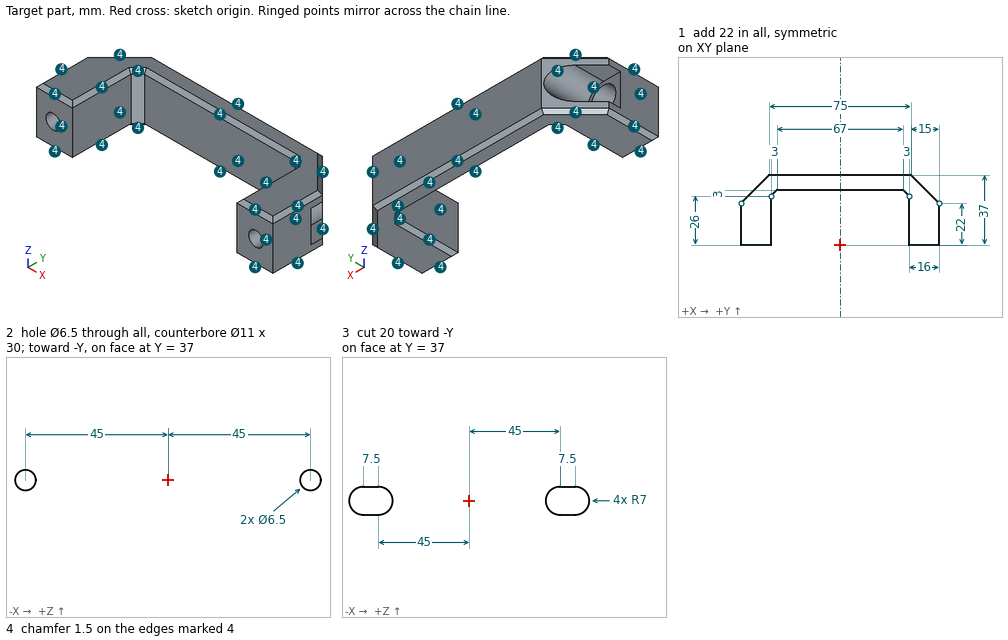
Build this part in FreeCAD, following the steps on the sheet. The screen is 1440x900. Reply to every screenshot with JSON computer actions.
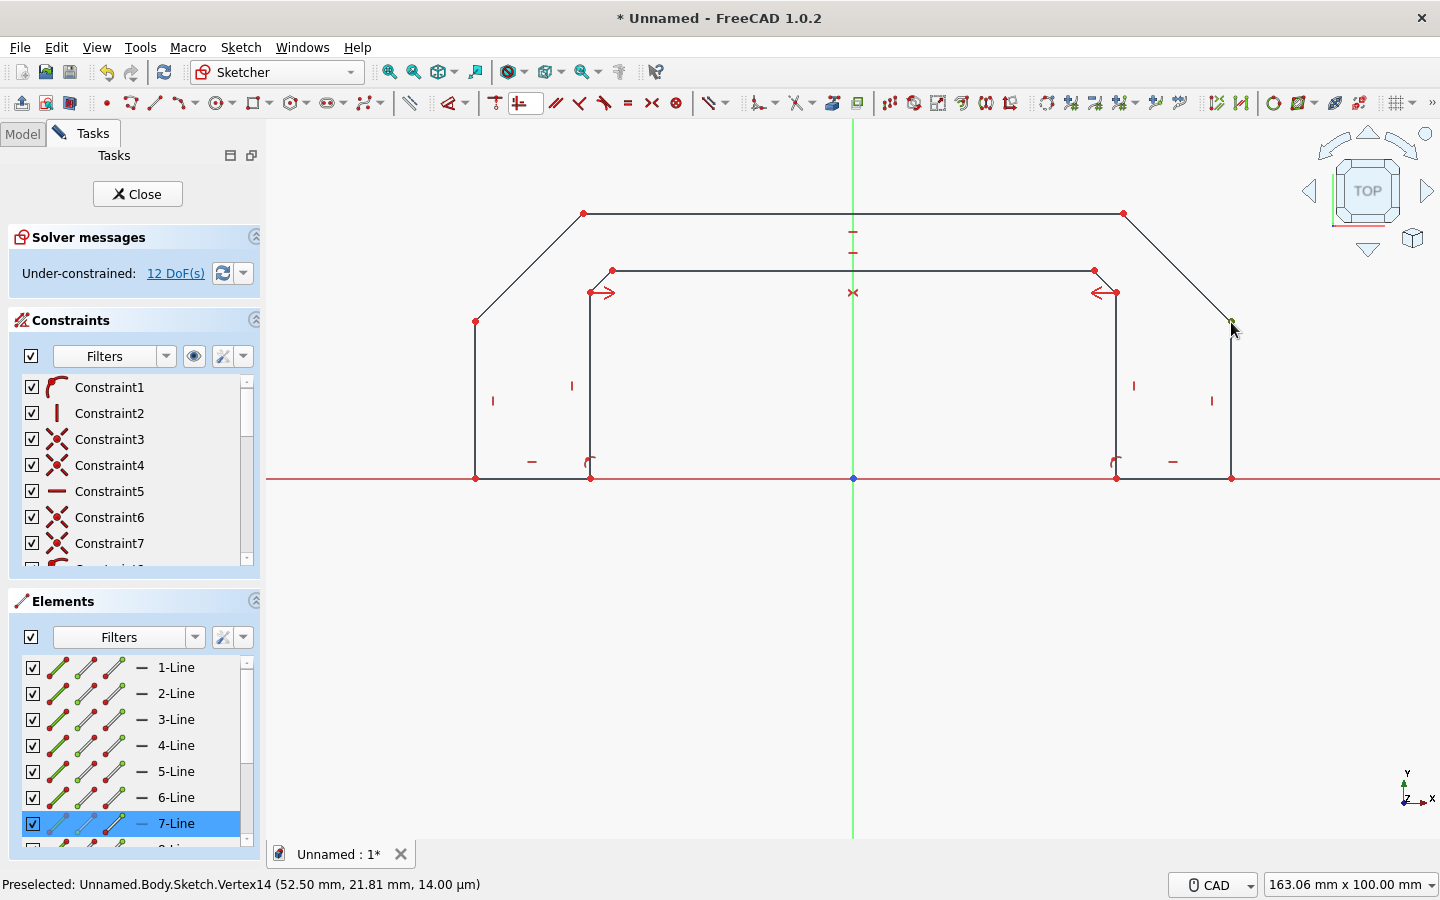
{"action": "left_click", "coordinate": [475, 322]}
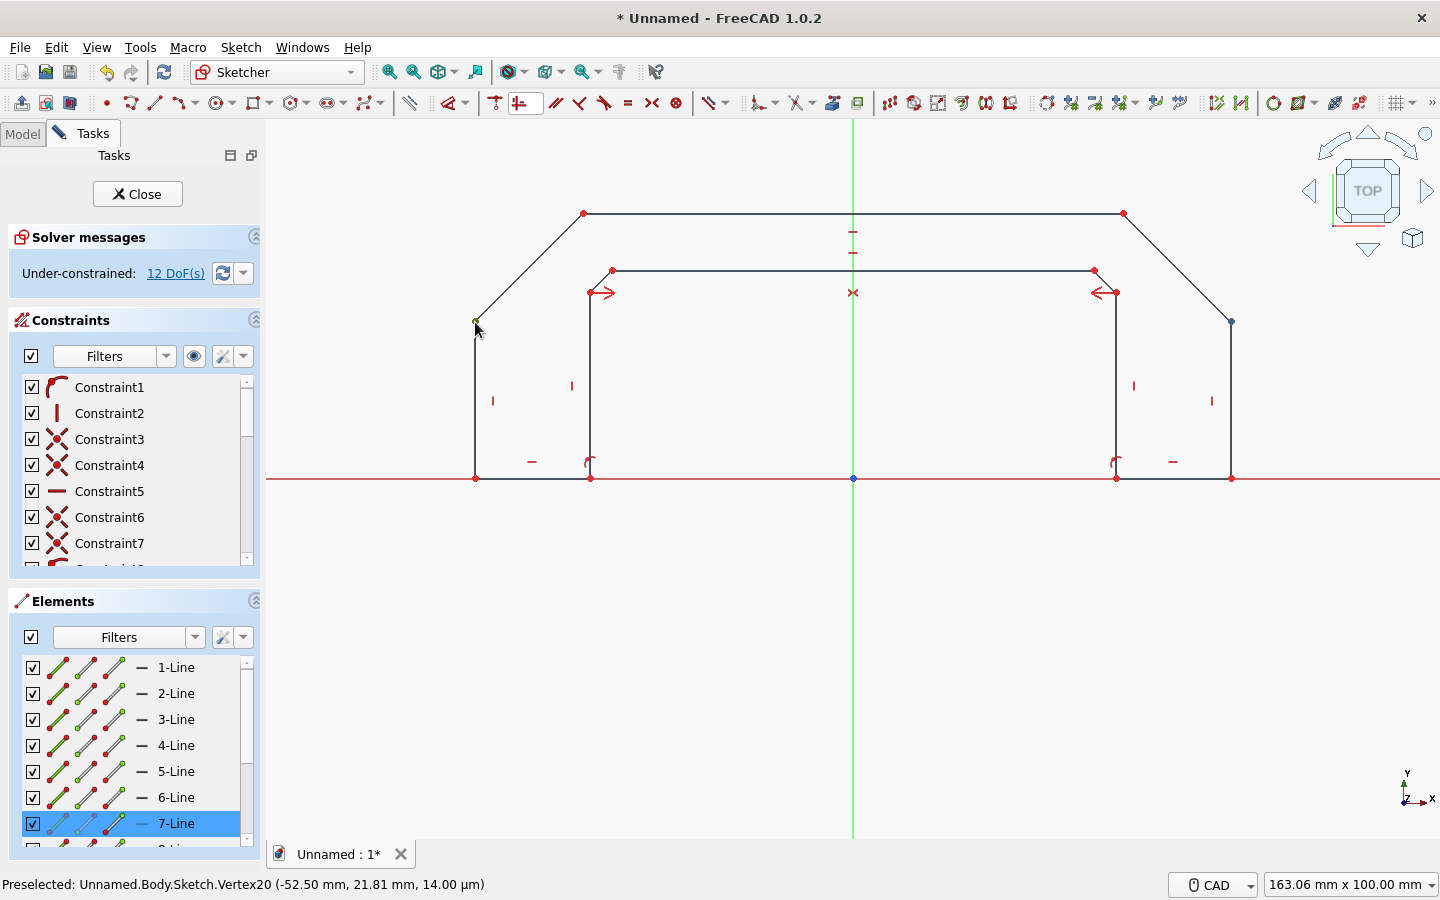
{"action": "left_click", "coordinate": [853, 764]}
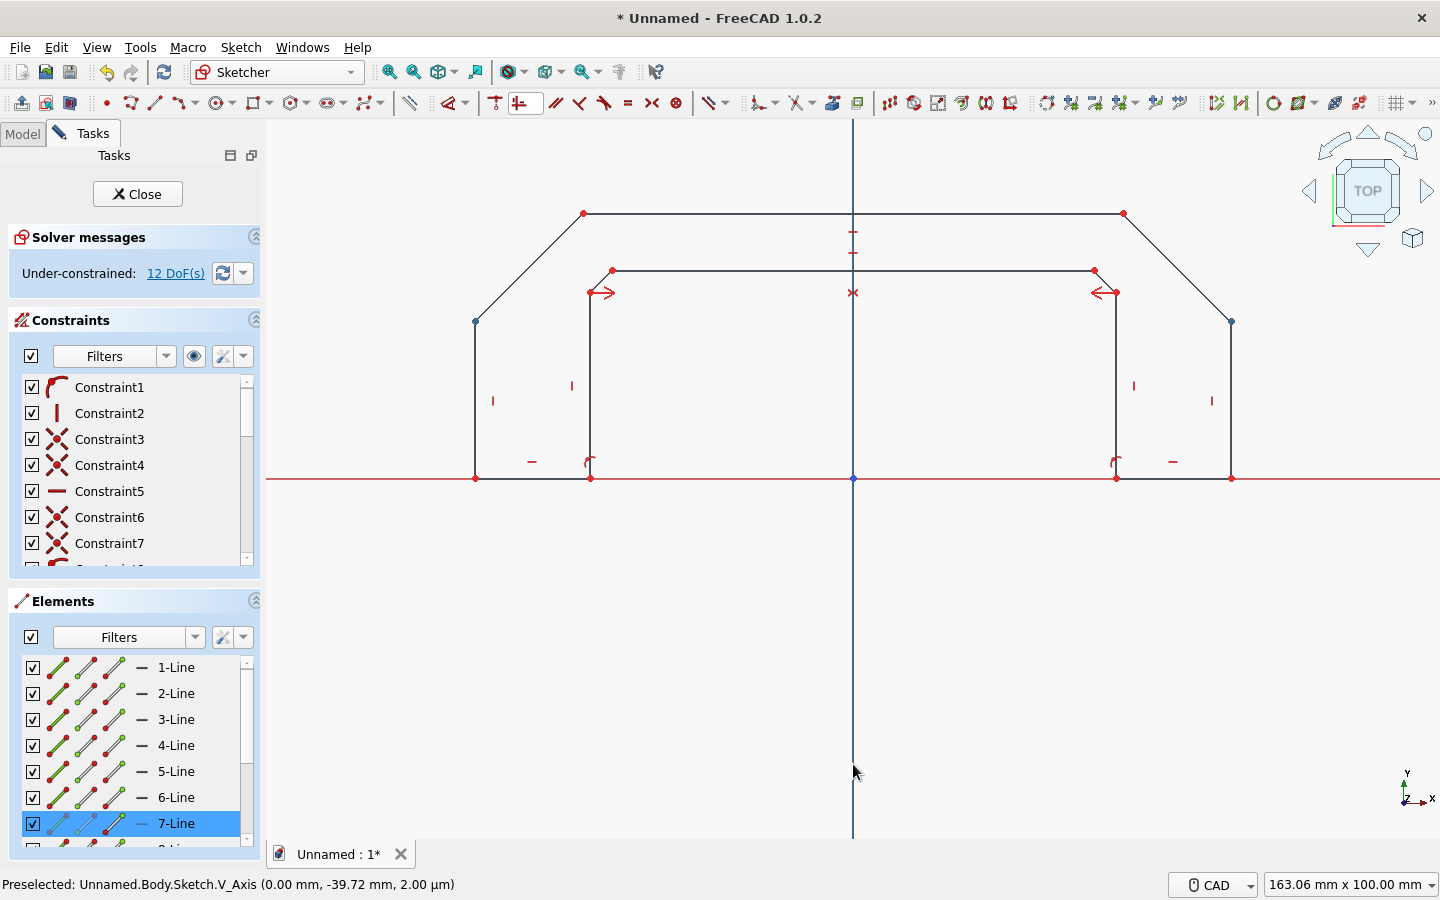
{"action": "left_click", "coordinate": [652, 104]}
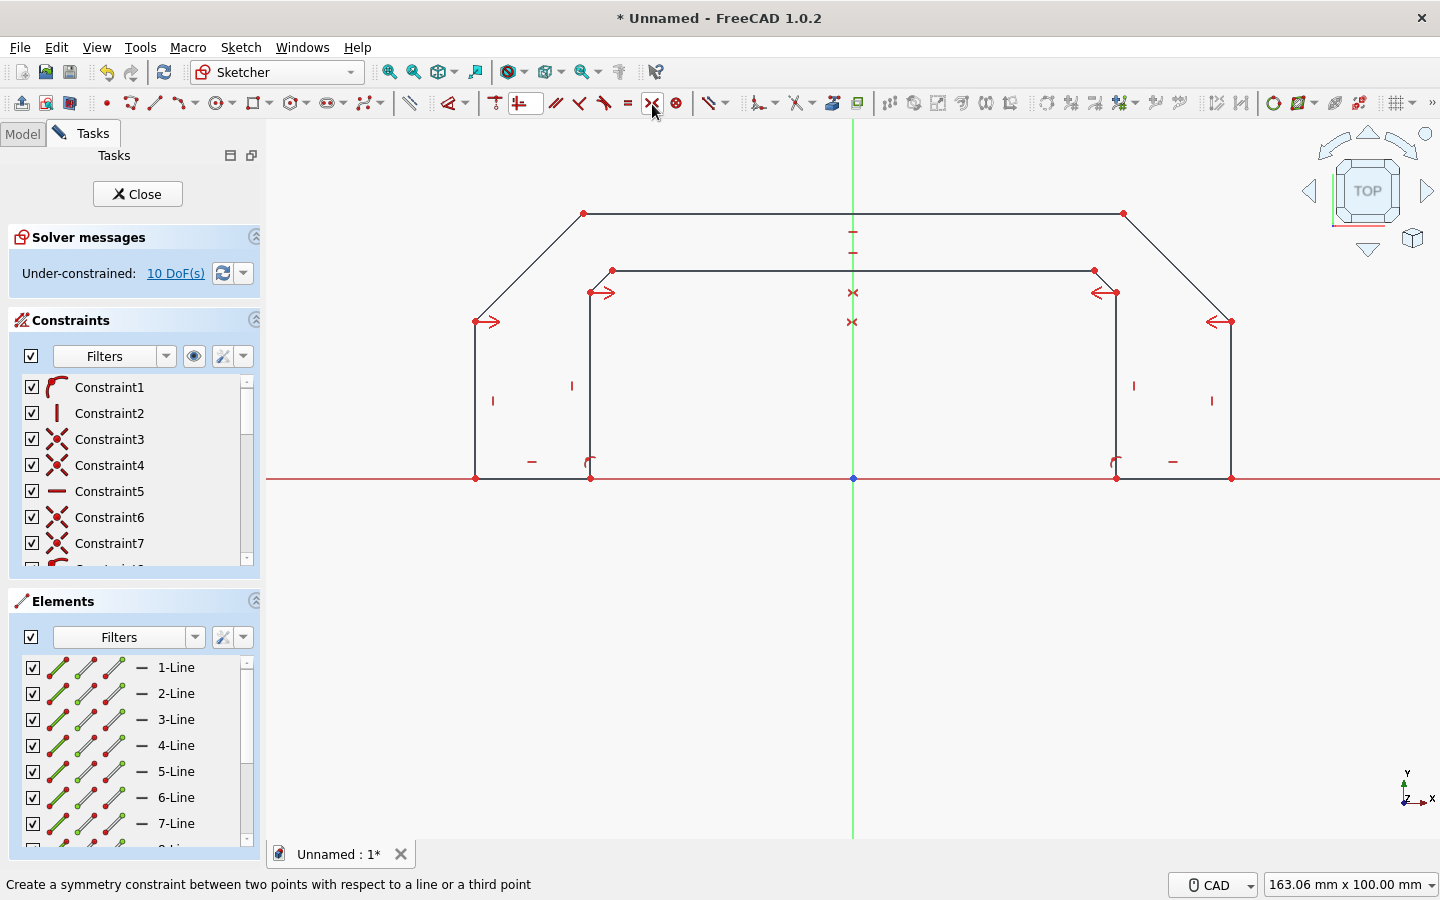
{"action": "left_click", "coordinate": [590, 423]}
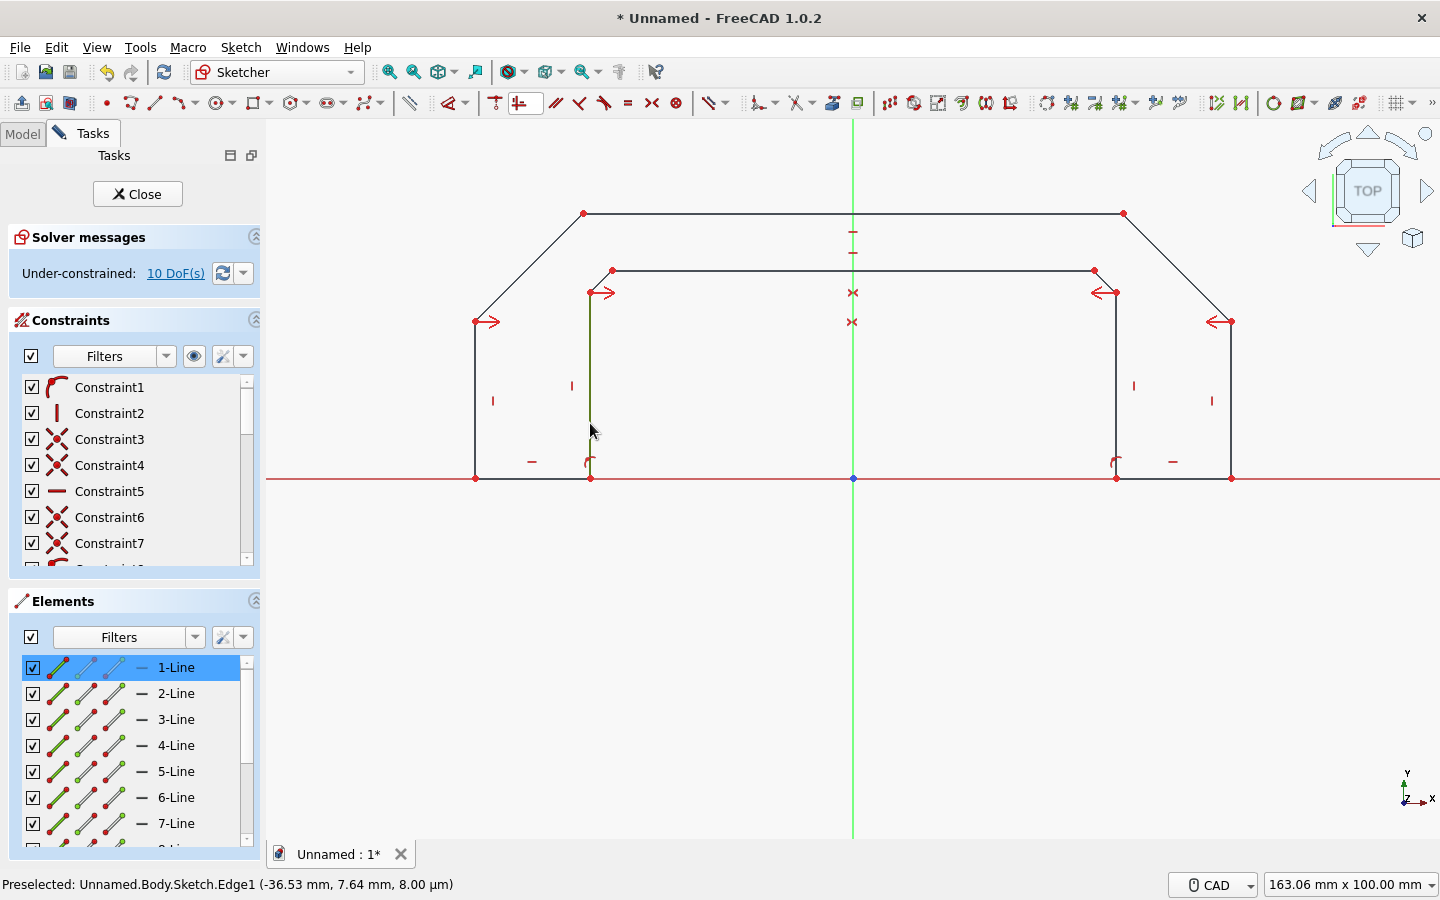
{"action": "left_click", "coordinate": [468, 104]}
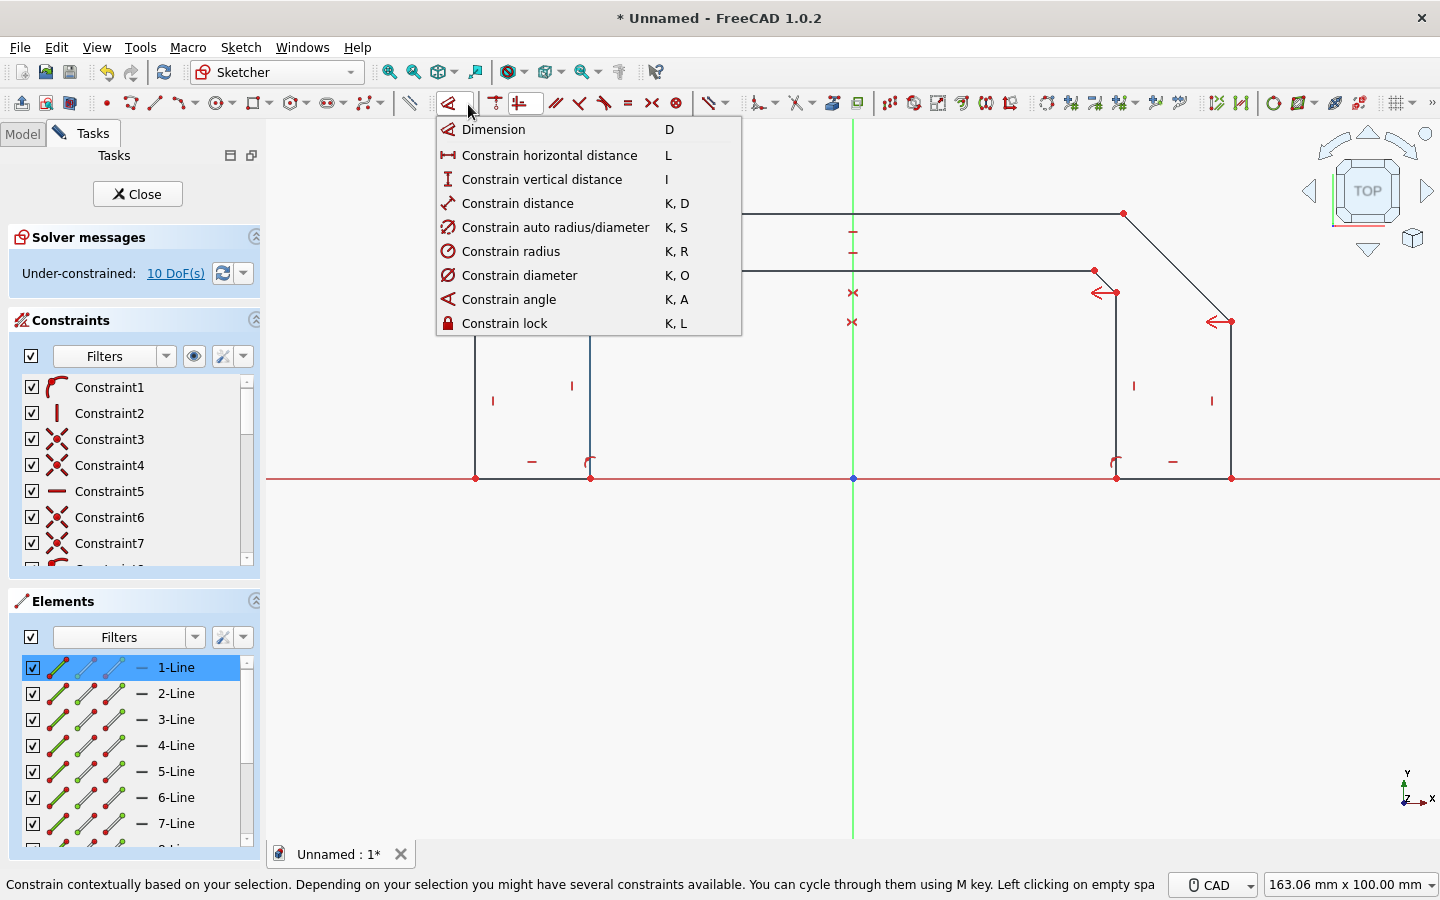
{"action": "left_click", "coordinate": [589, 179]}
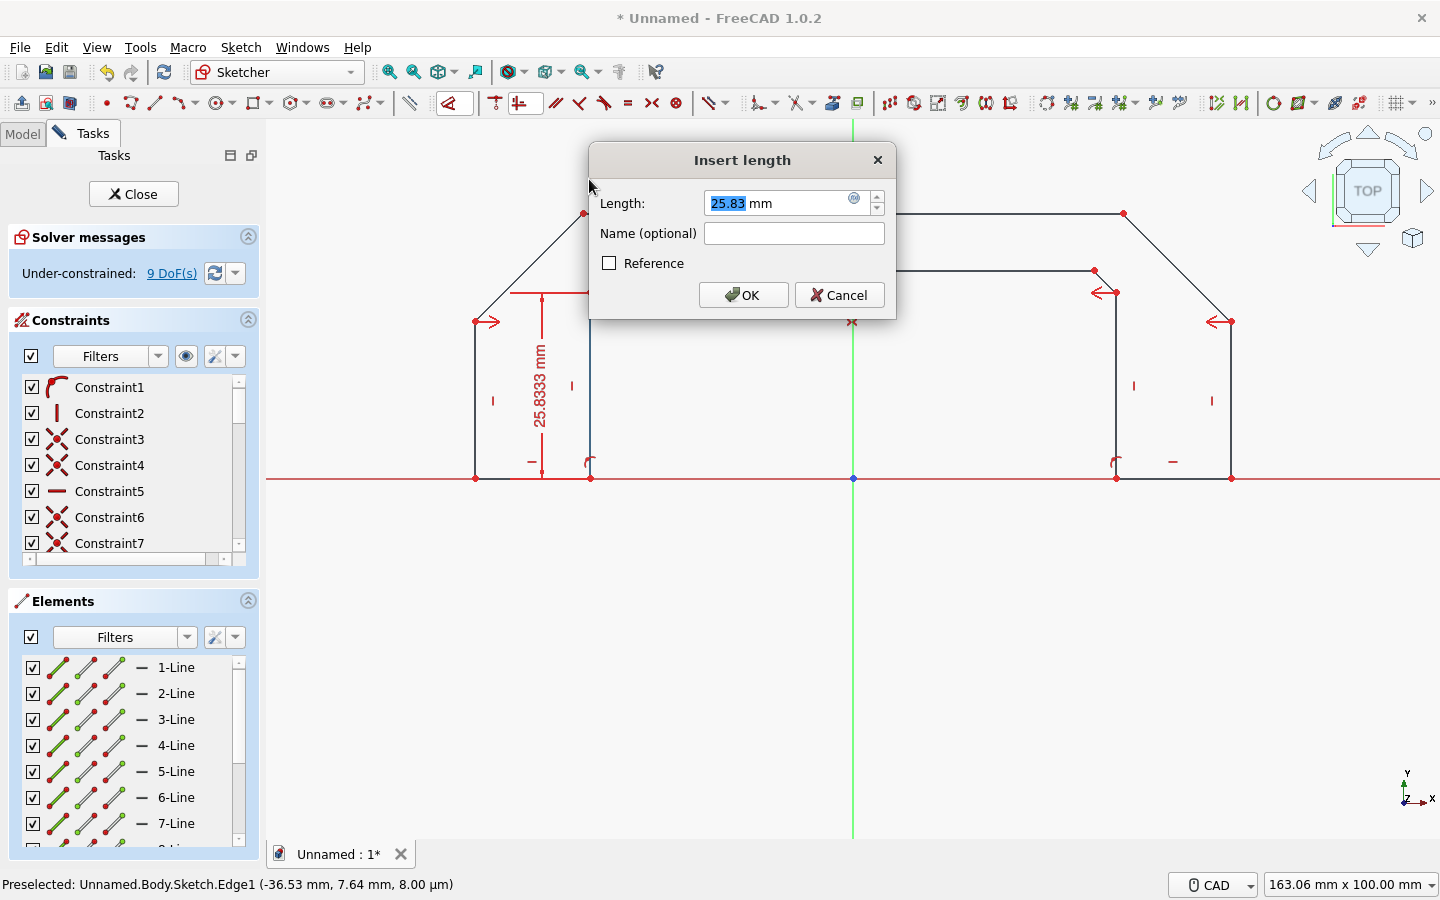
{"action": "type", "text": "26"}
{"action": "key", "text": "Return"}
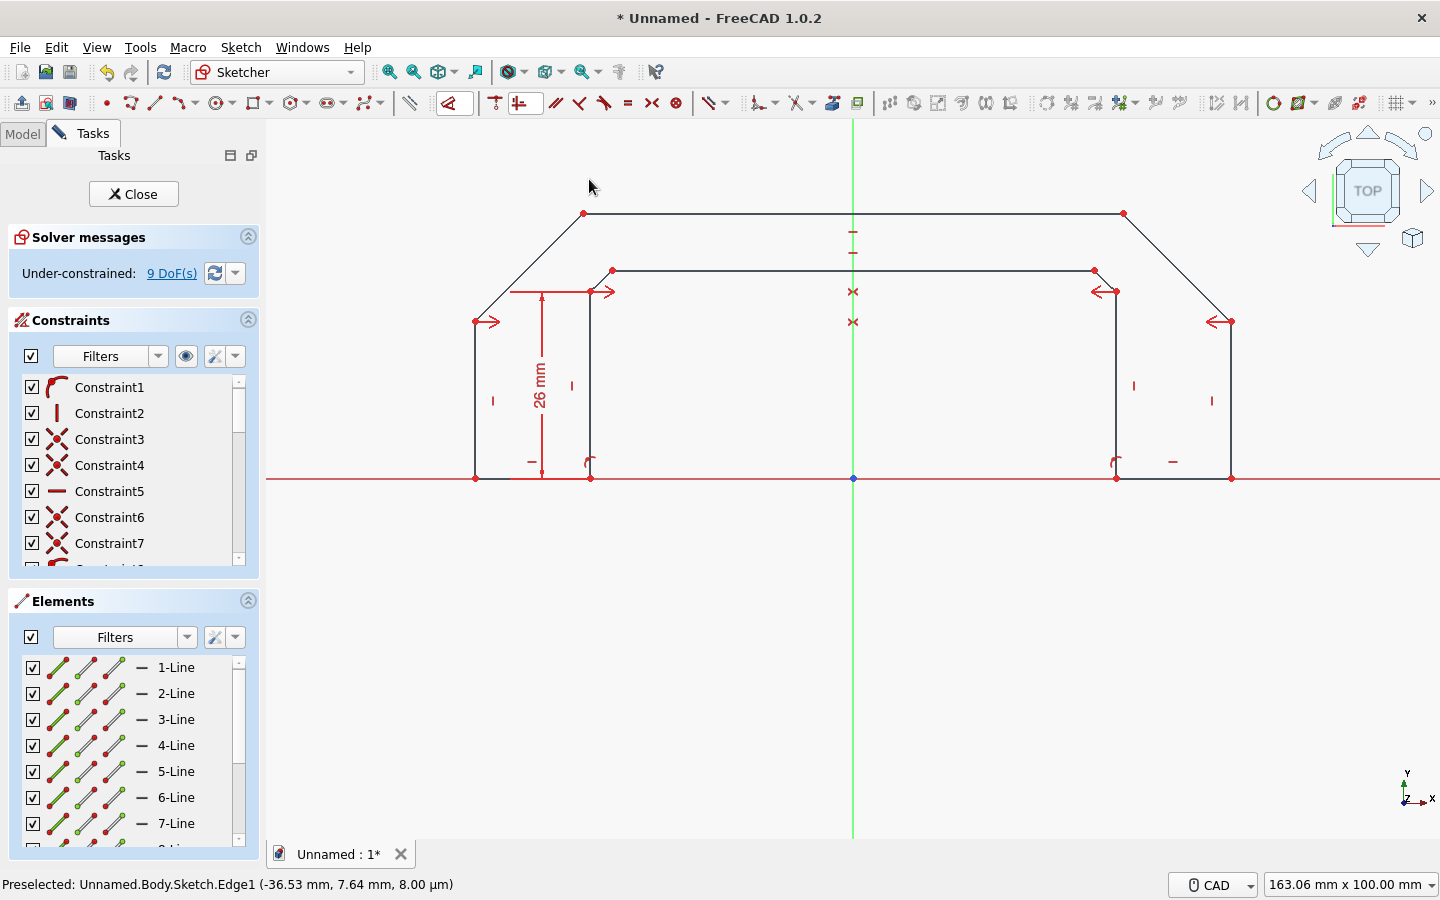
{"action": "left_click", "coordinate": [757, 271]}